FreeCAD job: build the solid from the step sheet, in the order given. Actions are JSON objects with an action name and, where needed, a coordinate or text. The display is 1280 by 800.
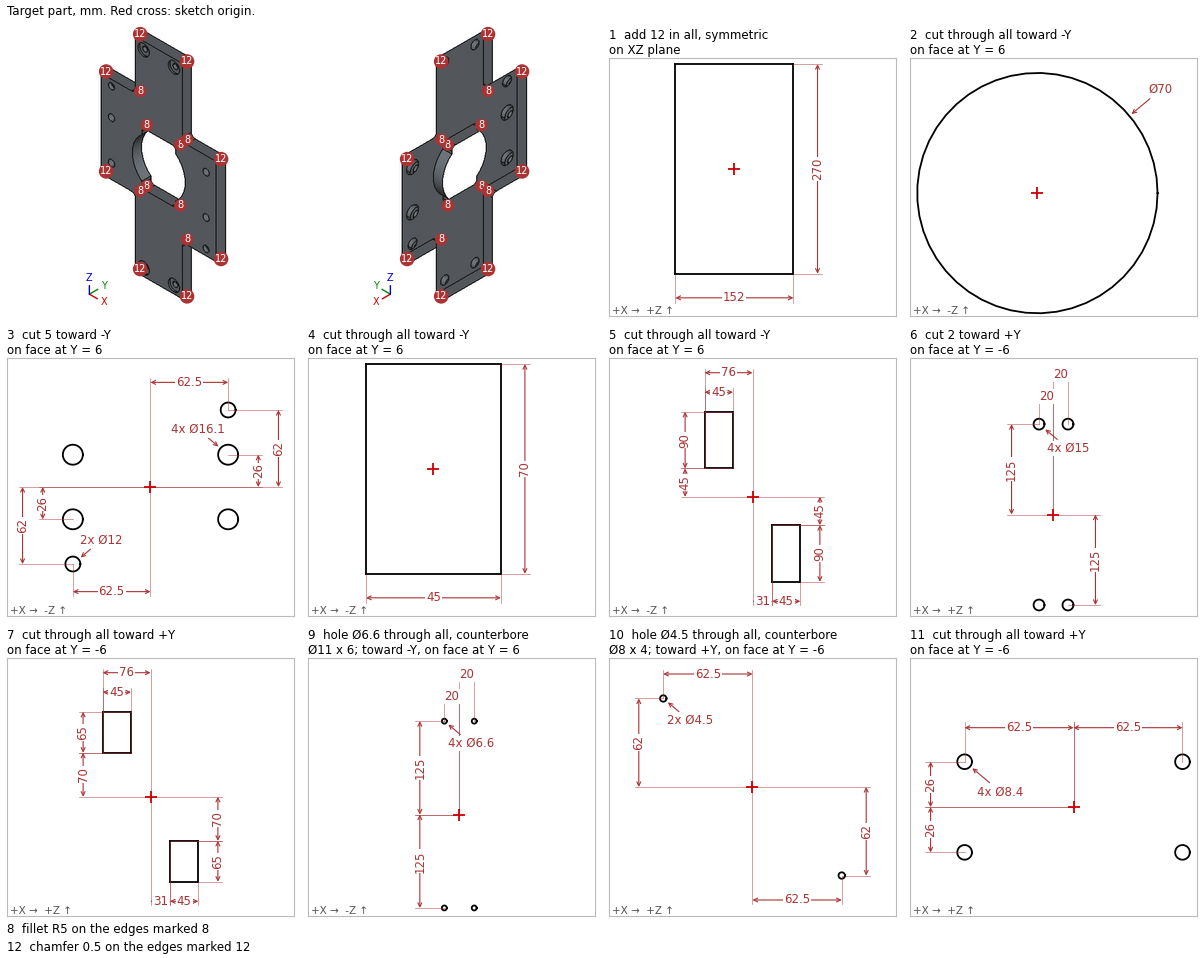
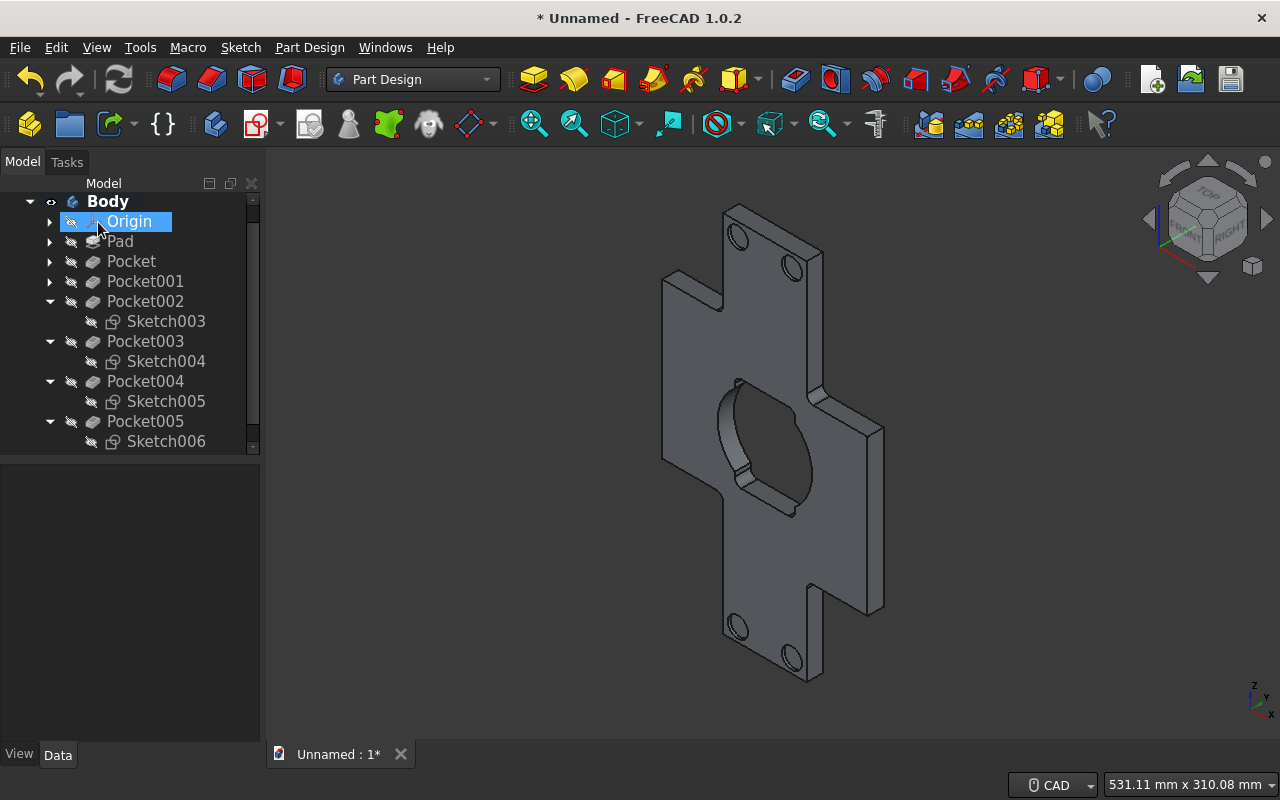
{"action": "key", "text": "4"}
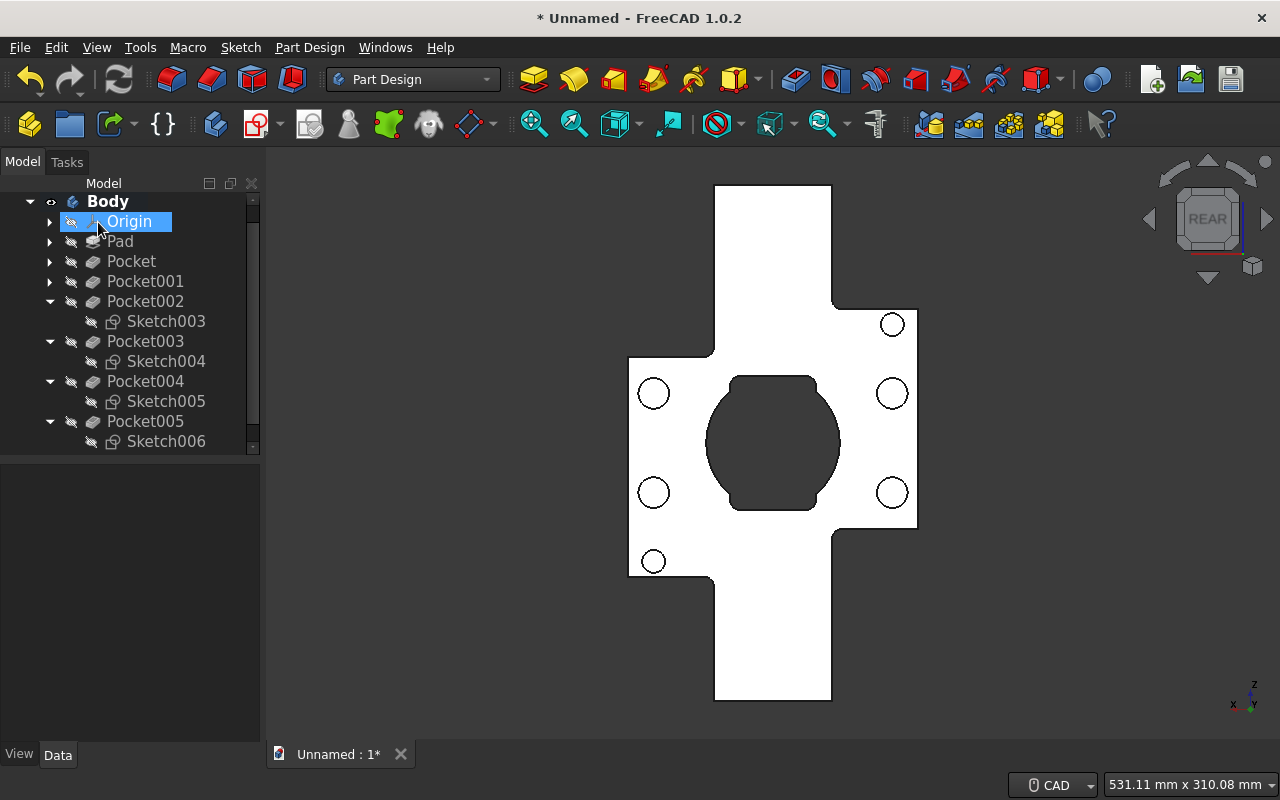
{"action": "left_click", "coordinate": [773, 295]}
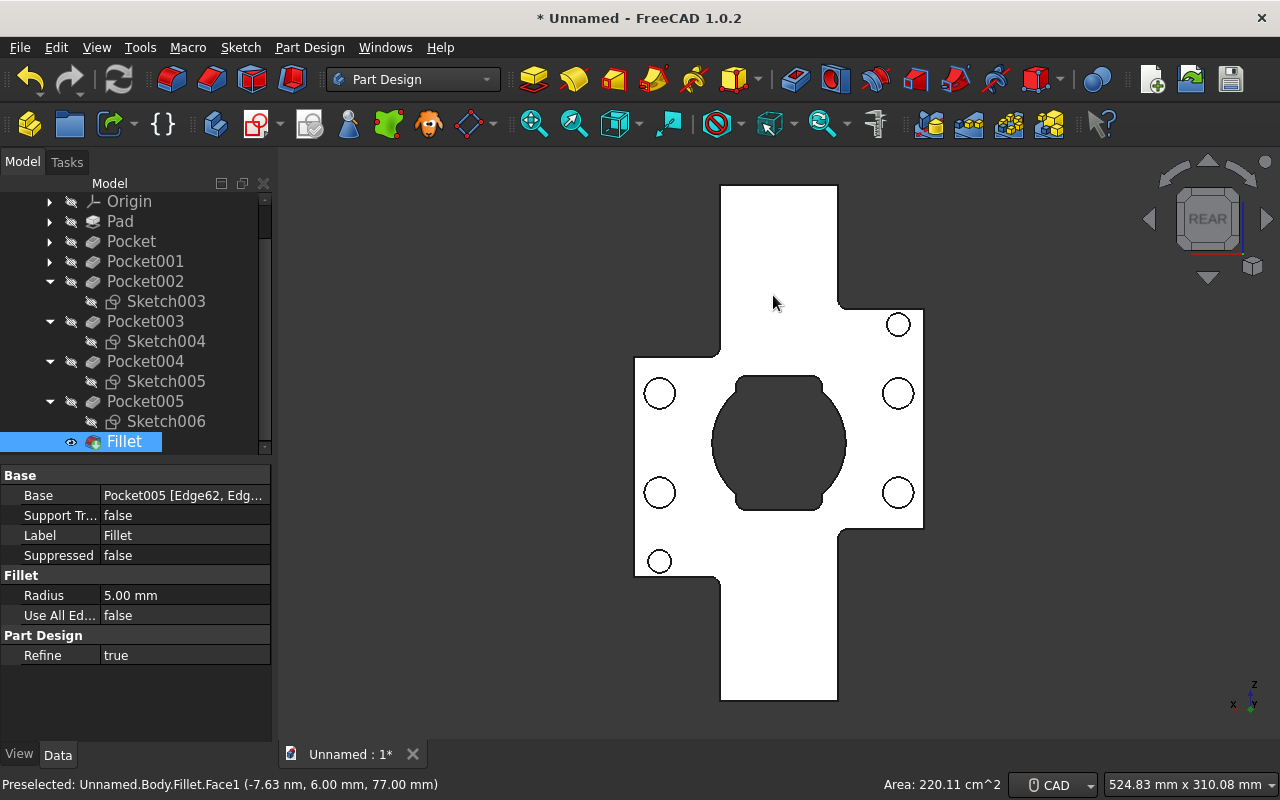
{"action": "left_click", "coordinate": [256, 124]}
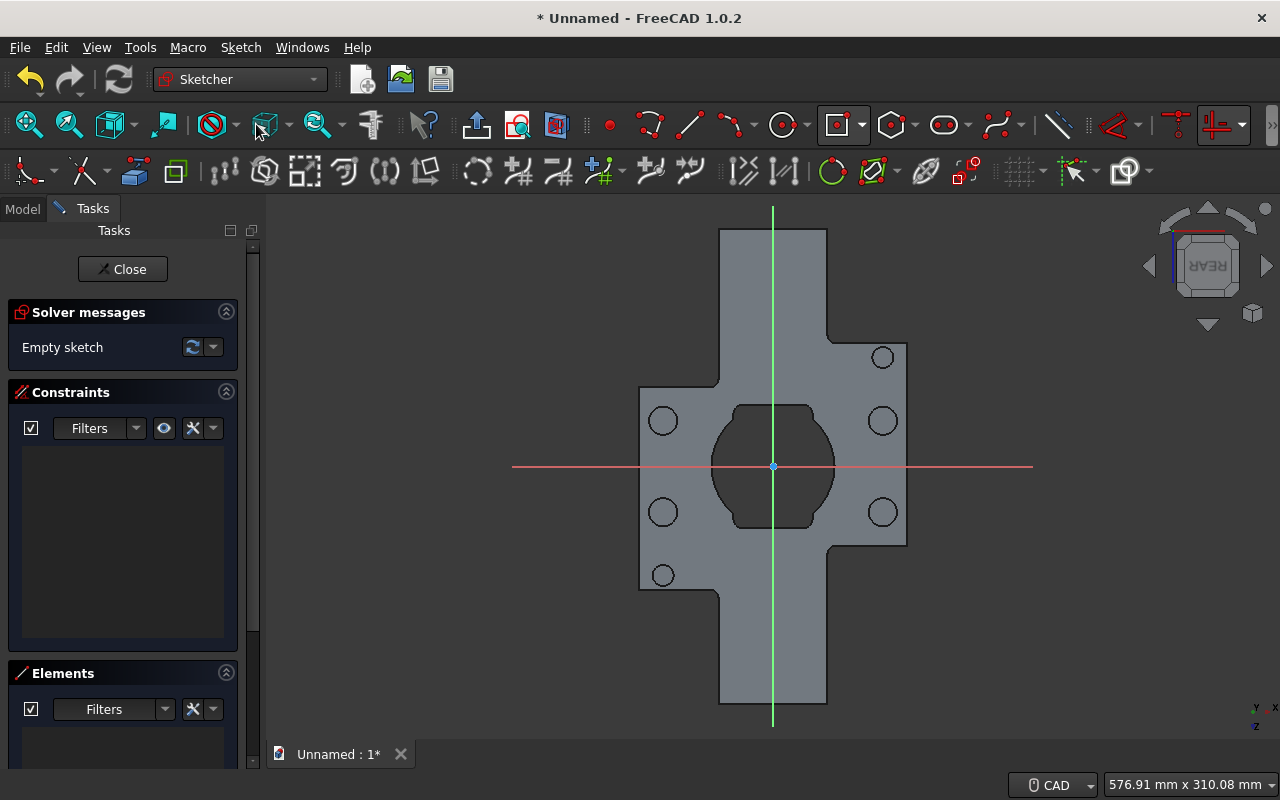
{"action": "scroll", "coordinate": [395, 466], "scroll_direction": "down", "scroll_amount": 1}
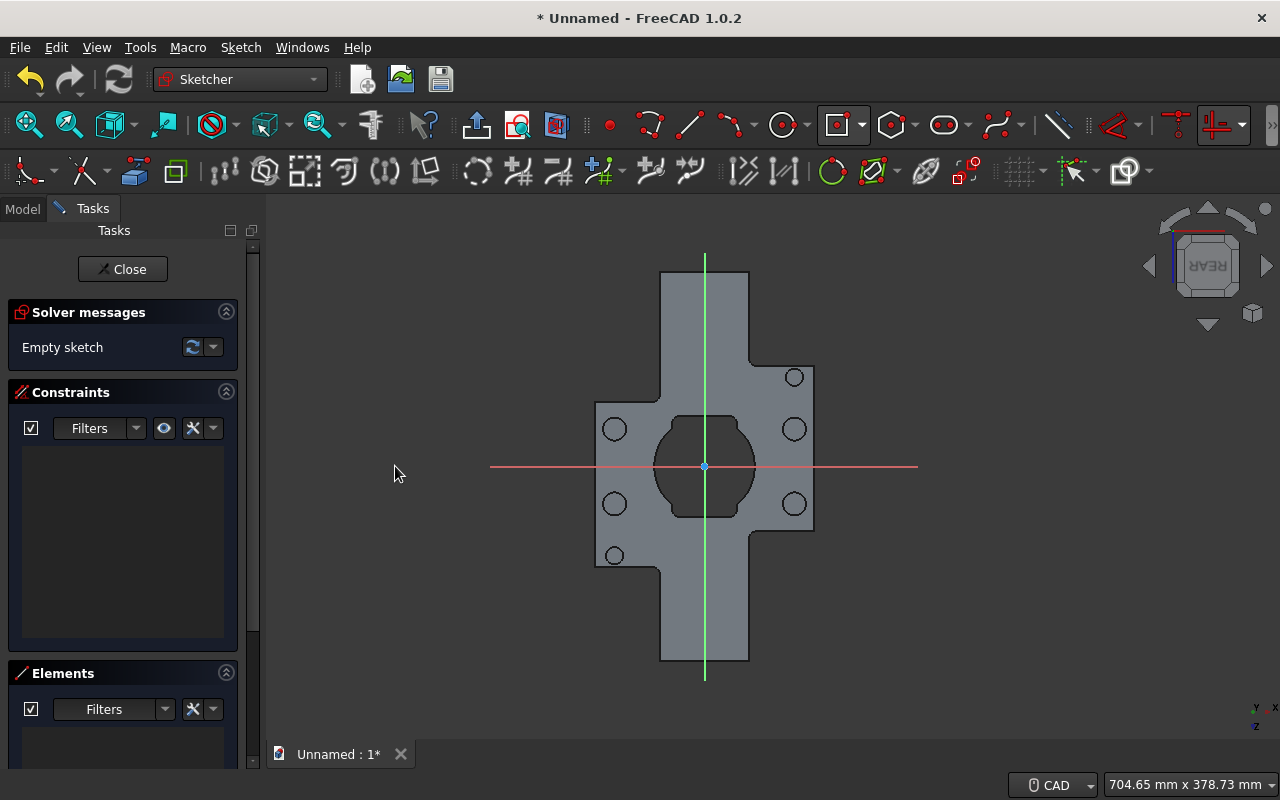
{"action": "left_click", "coordinate": [784, 126]}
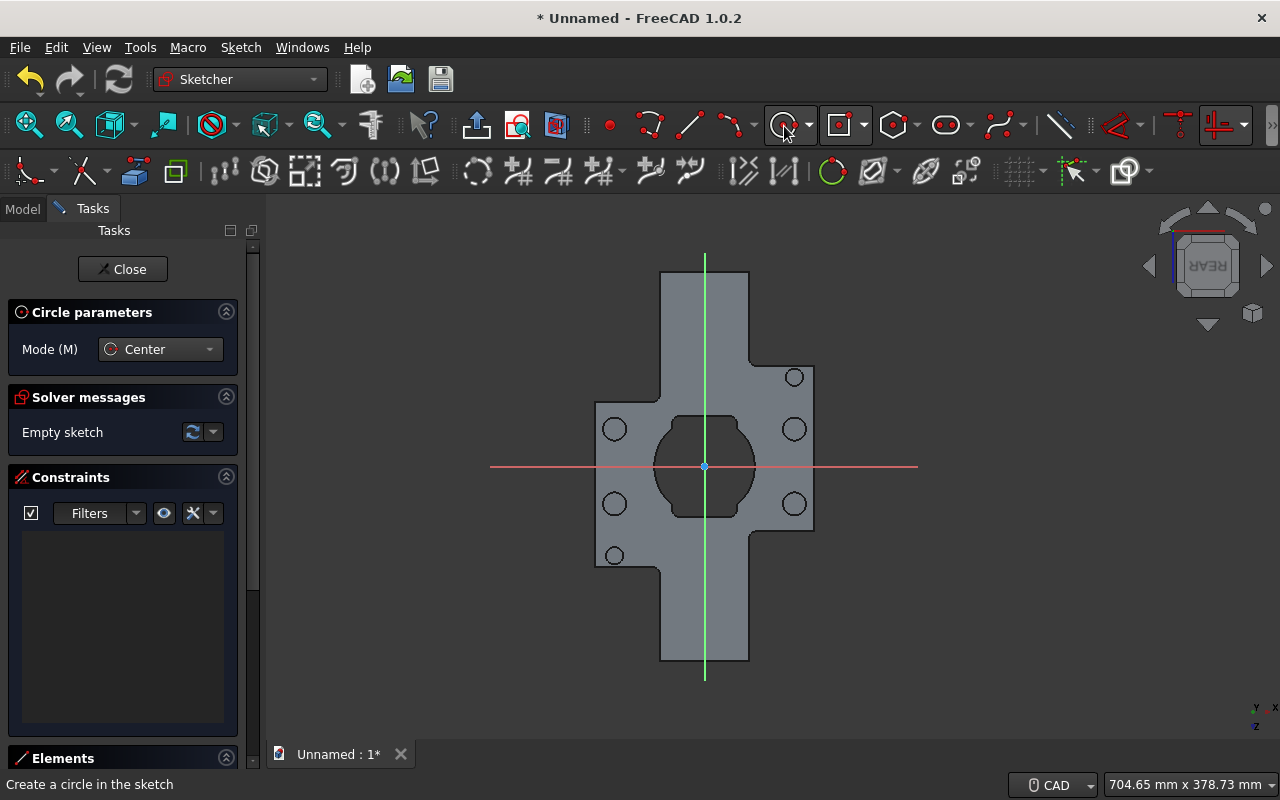
{"action": "scroll", "coordinate": [676, 287], "scroll_direction": "up", "scroll_amount": 8}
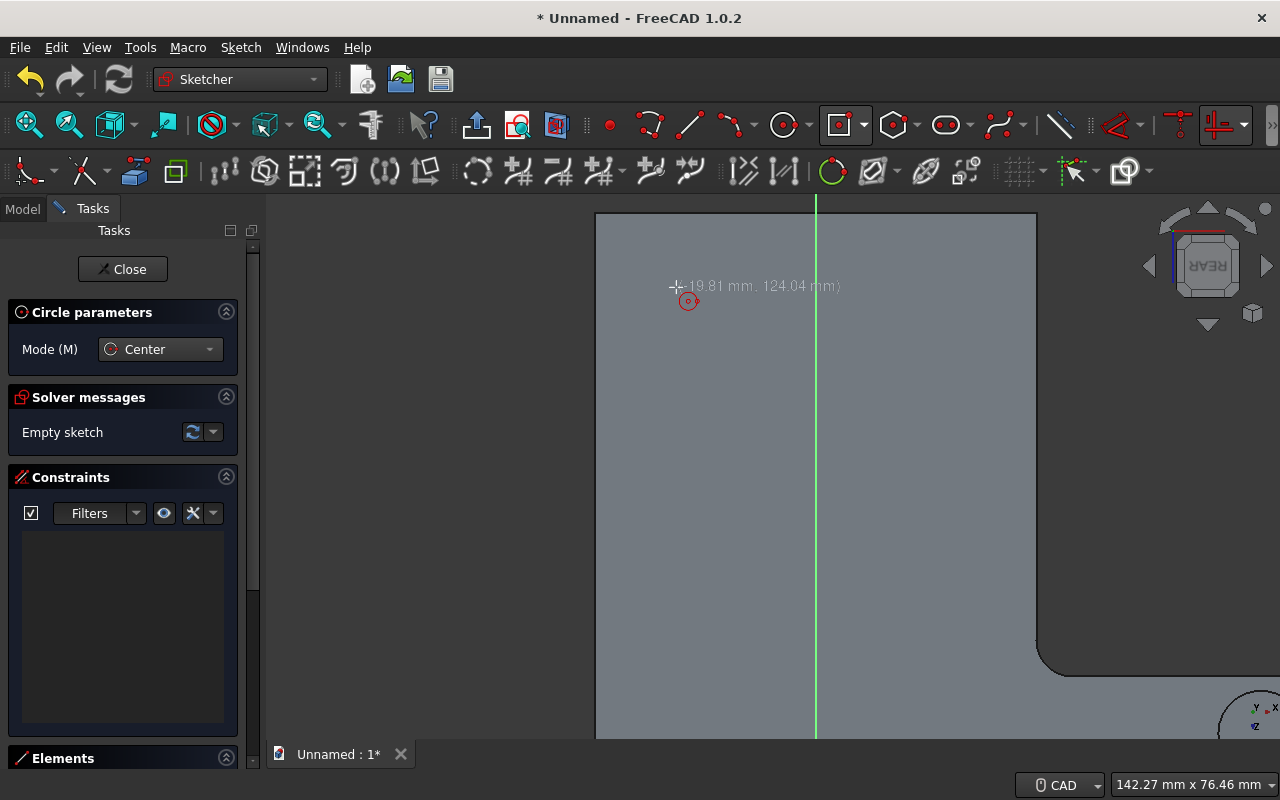
{"action": "scroll", "coordinate": [676, 287], "scroll_direction": "down", "scroll_amount": 8}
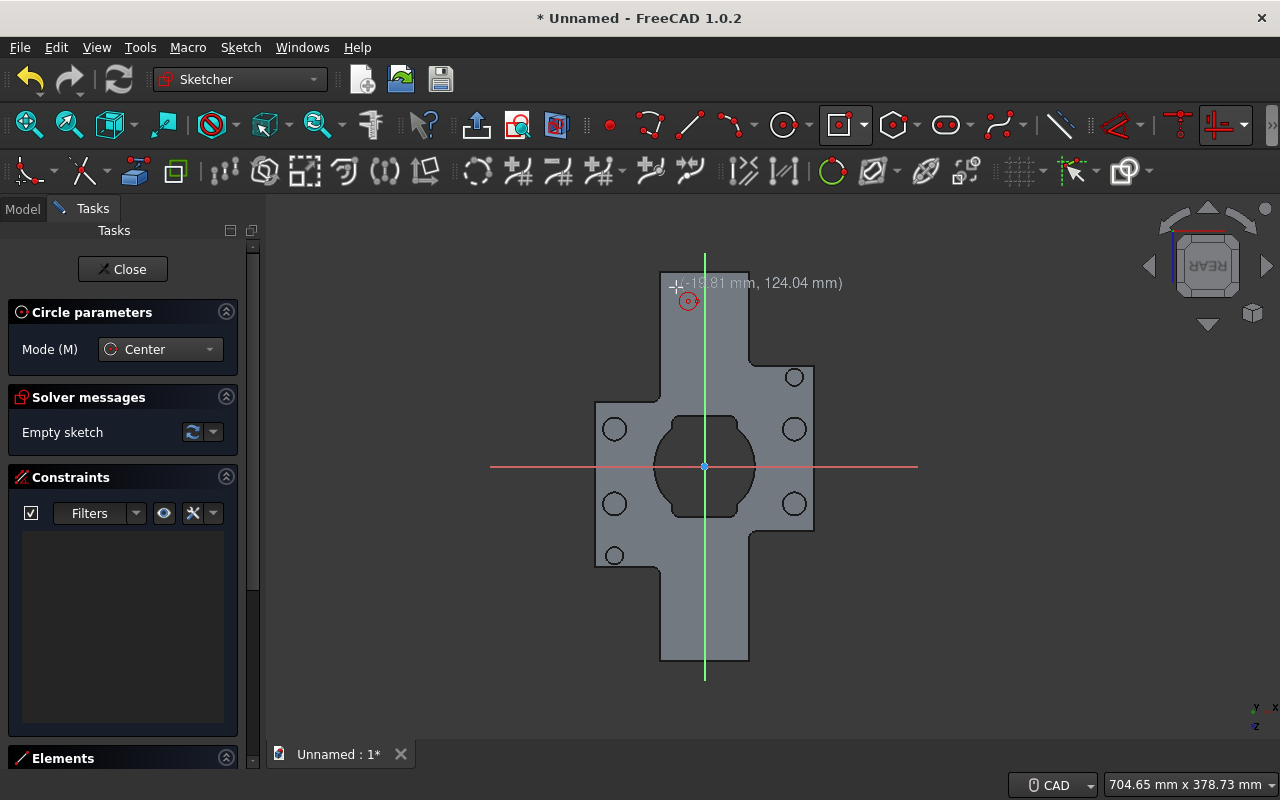
{"action": "left_click", "coordinate": [676, 287]}
{"action": "mouse_move", "coordinate": [679, 283]}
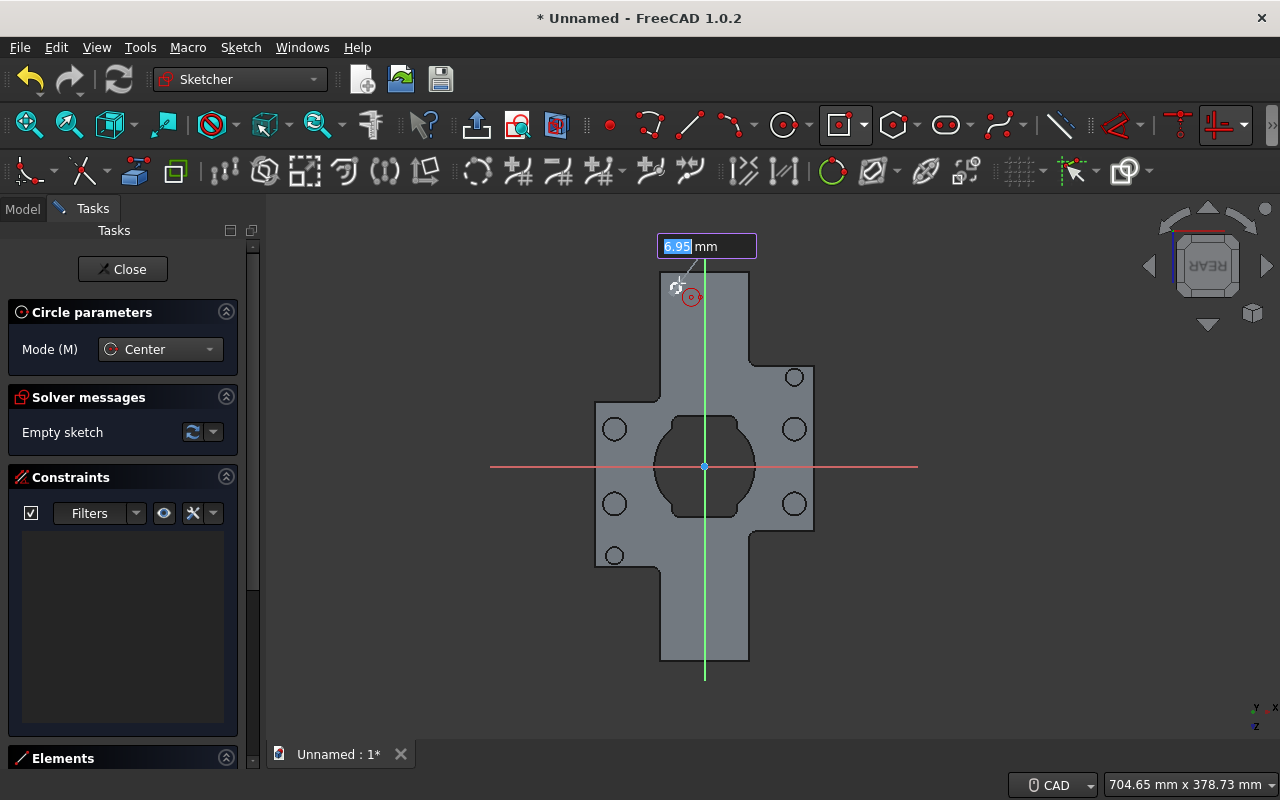
{"action": "type", "text": "6.6"}
{"action": "key", "text": "Return"}